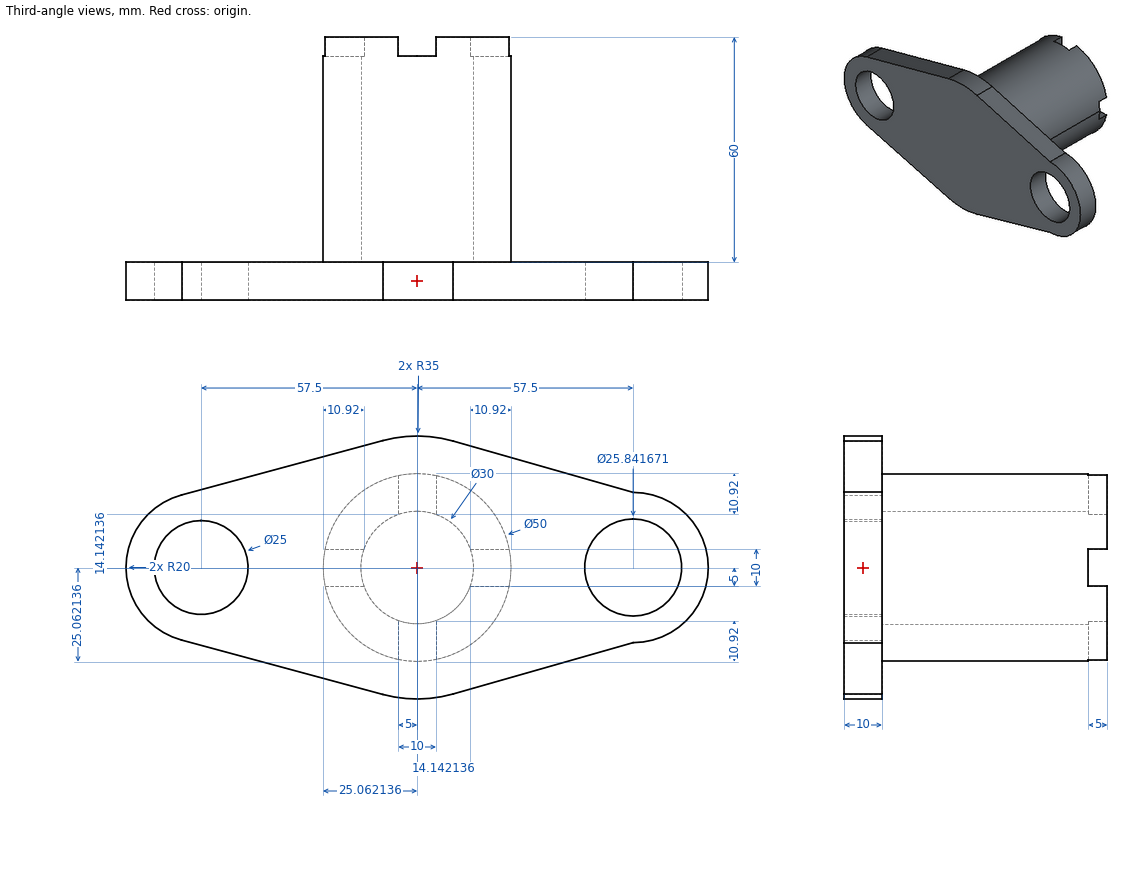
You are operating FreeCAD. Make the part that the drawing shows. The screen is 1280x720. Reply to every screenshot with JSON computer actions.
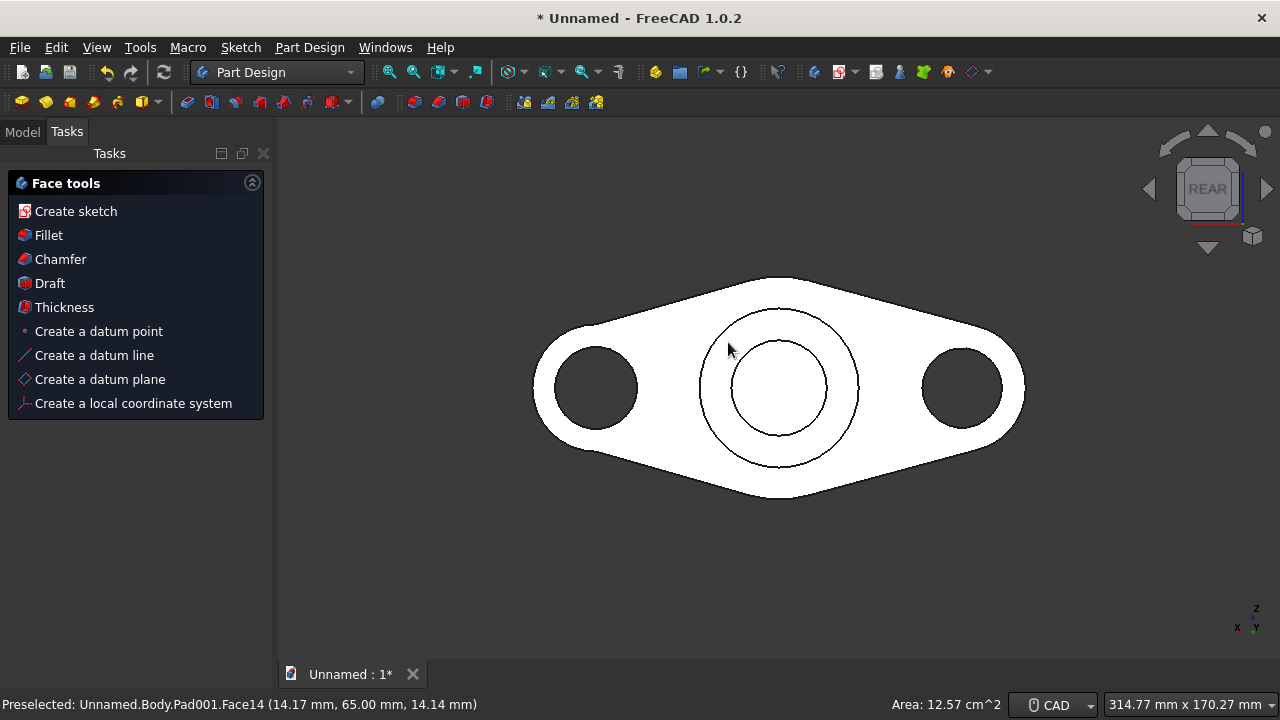
{"action": "left_click", "coordinate": [840, 72]}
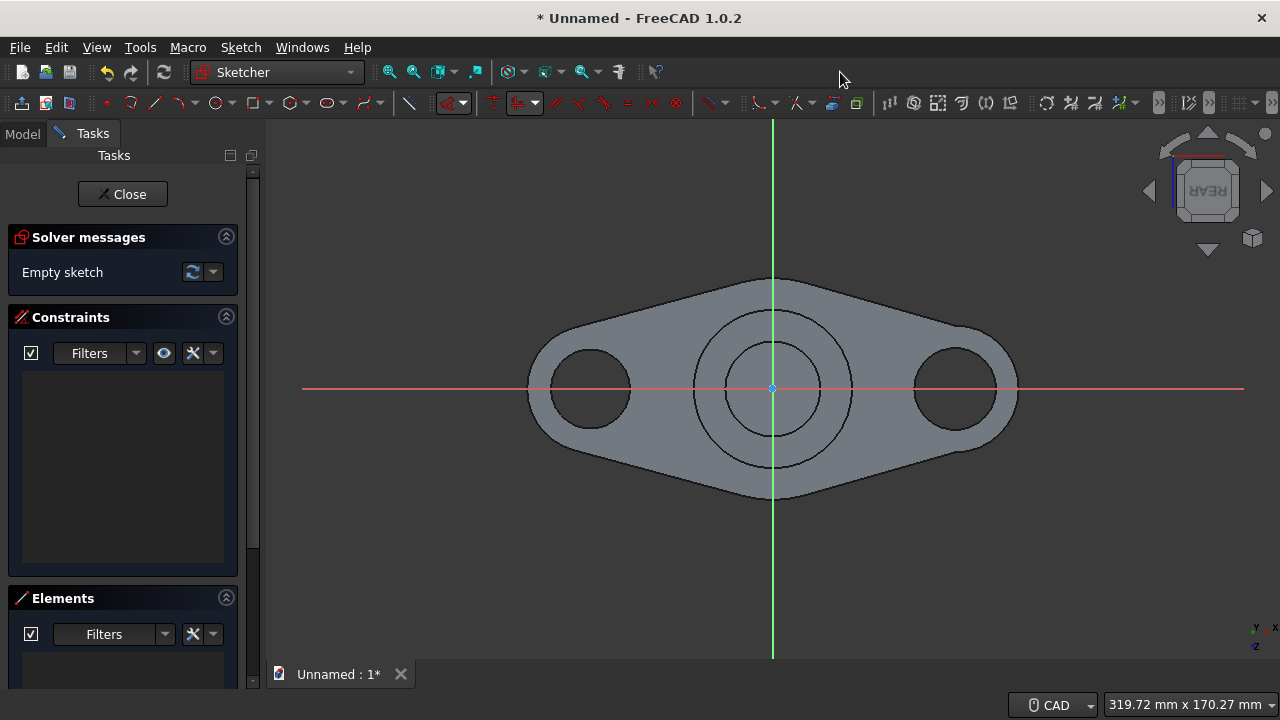
{"action": "scroll", "coordinate": [829, 389], "scroll_direction": "up", "scroll_amount": 4}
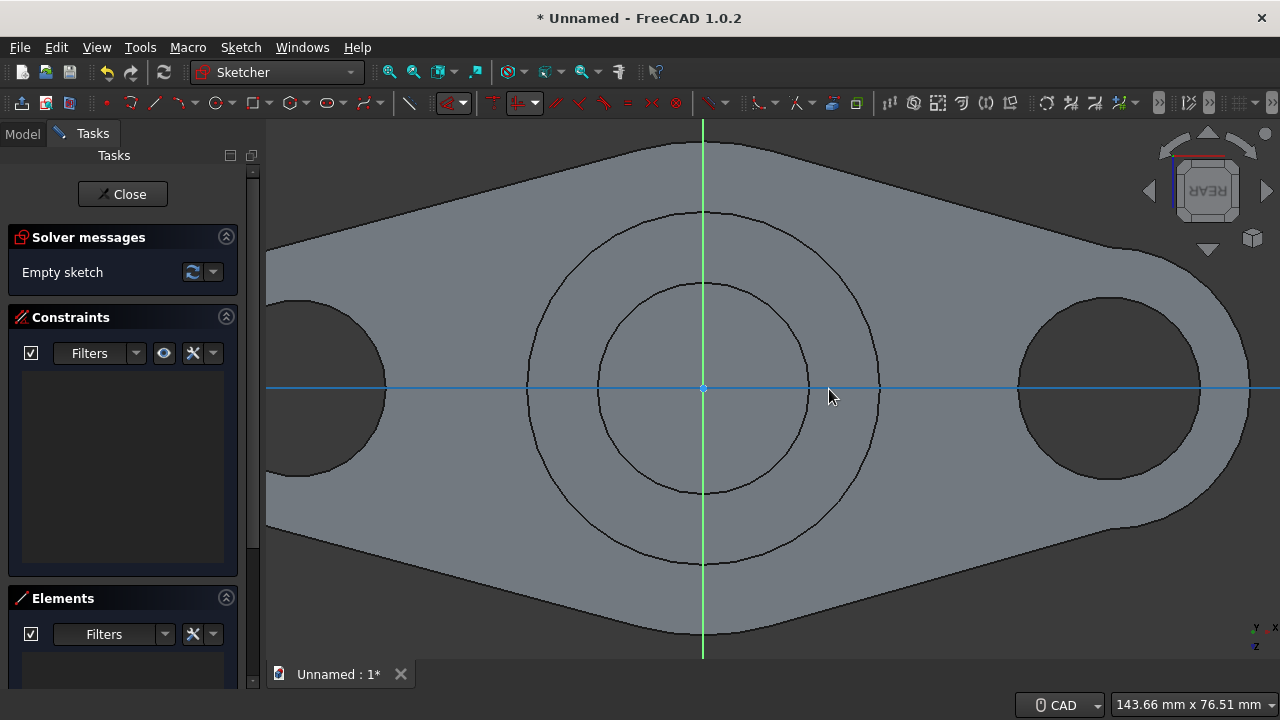
{"action": "left_click", "coordinate": [254, 104]}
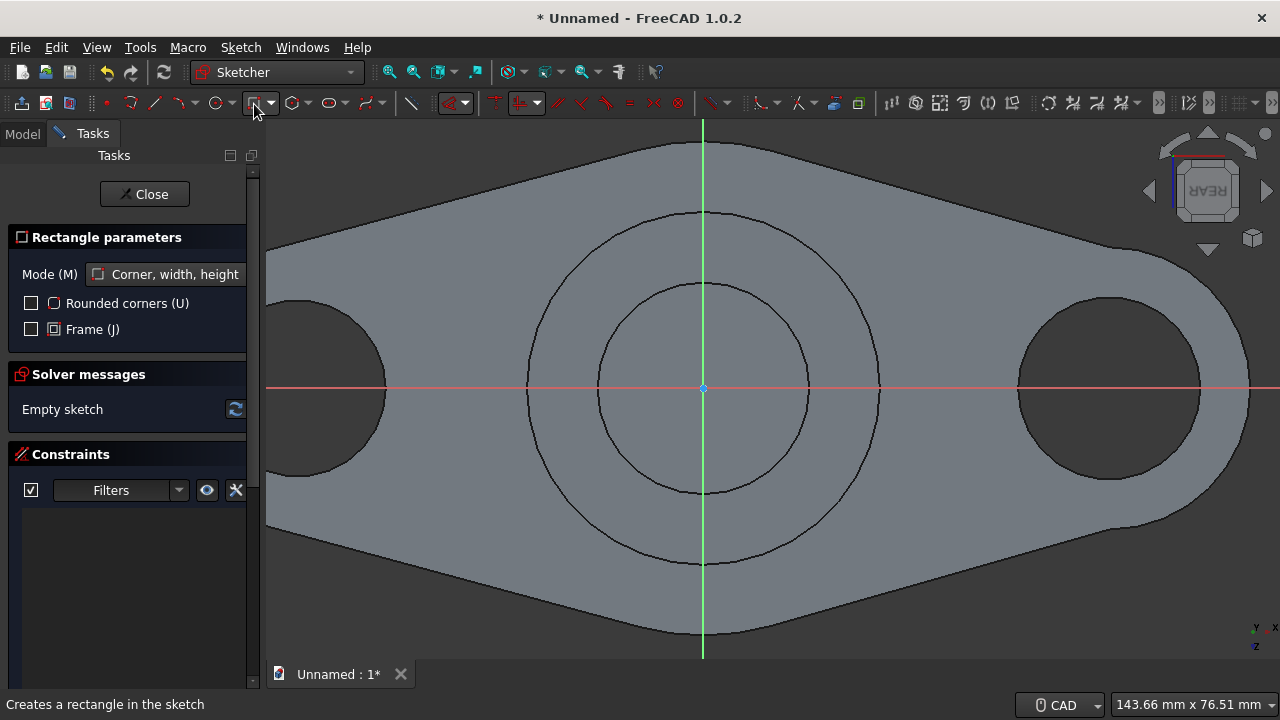
{"action": "left_click", "coordinate": [668, 211]}
{"action": "mouse_move", "coordinate": [739, 289]}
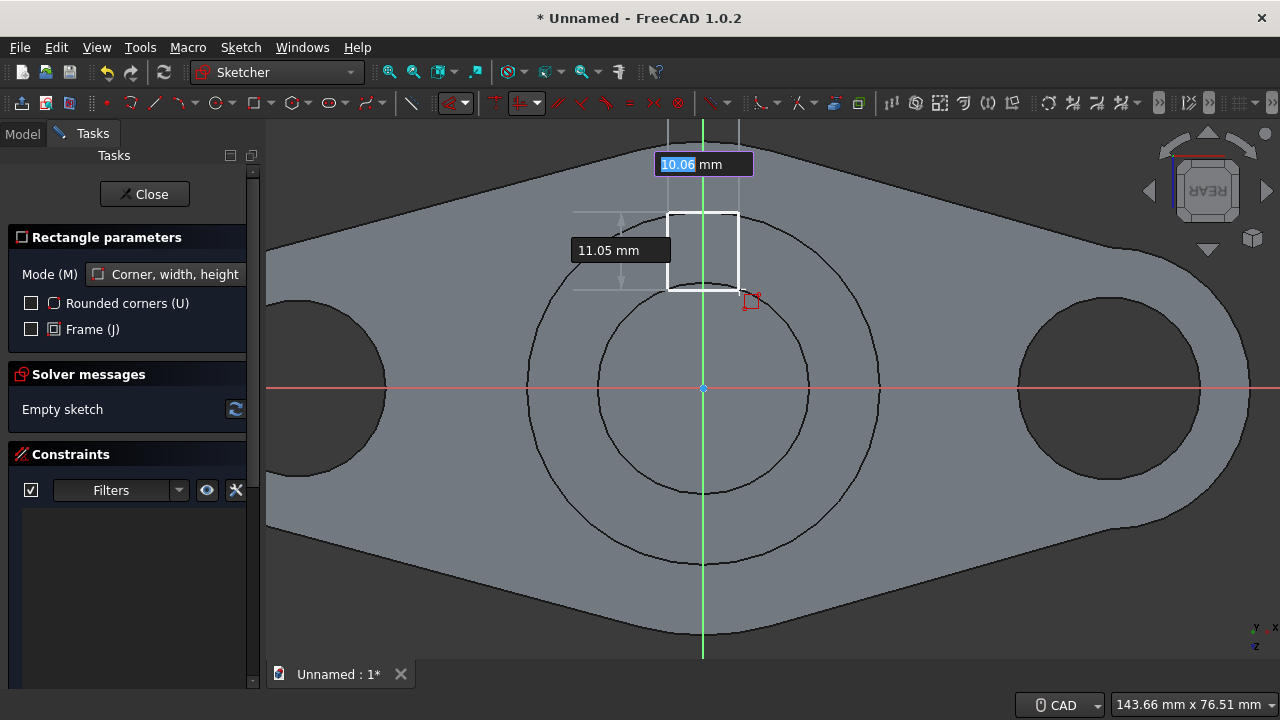
{"action": "type", "text": "10"}
{"action": "key", "text": "Tab"}
{"action": "type", "text": "10.92"}
{"action": "key", "text": "Return"}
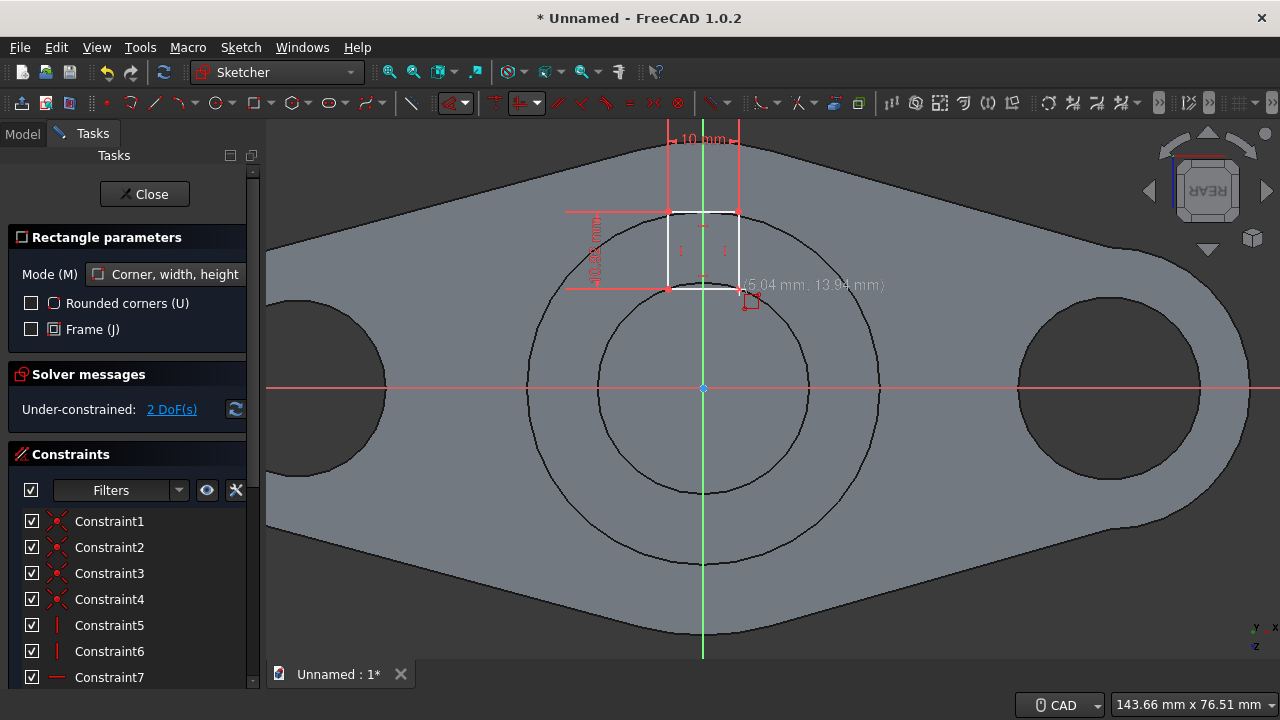
{"action": "left_click", "coordinate": [803, 353]}
{"action": "mouse_move", "coordinate": [880, 424]}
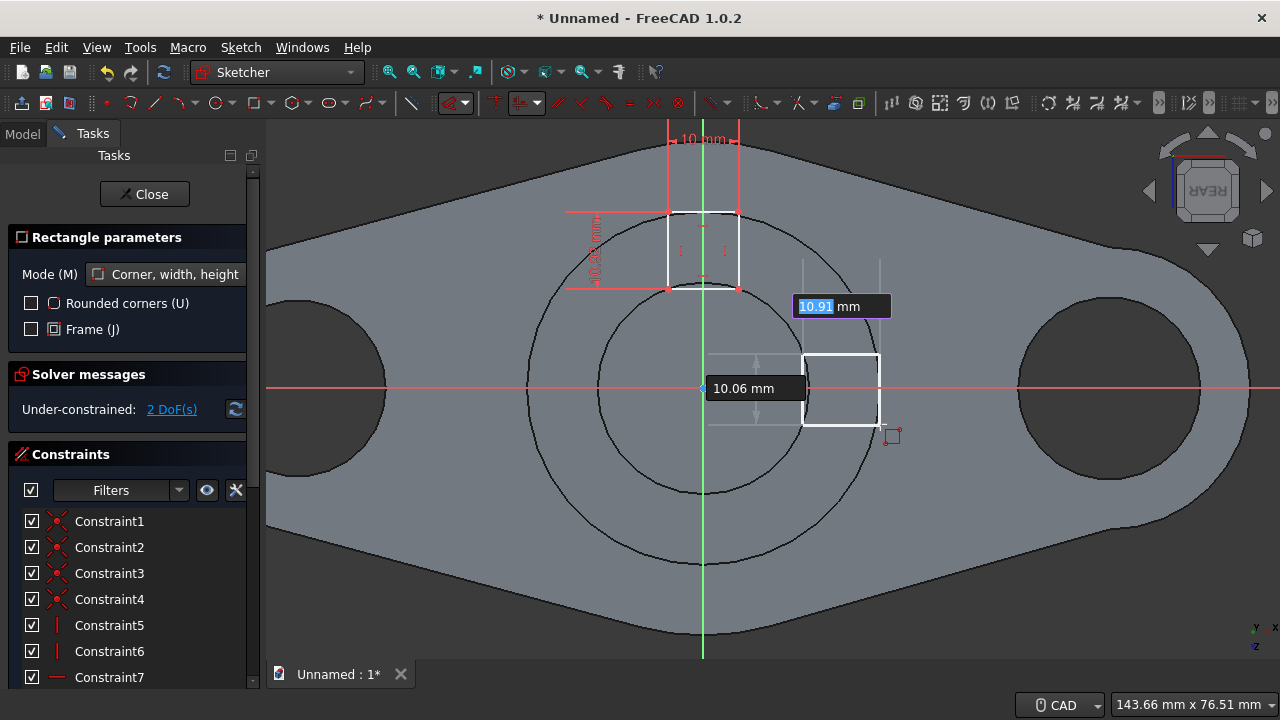
{"action": "type", "text": "10.92"}
{"action": "key", "text": "Tab"}
{"action": "type", "text": "10"}
{"action": "key", "text": "Return"}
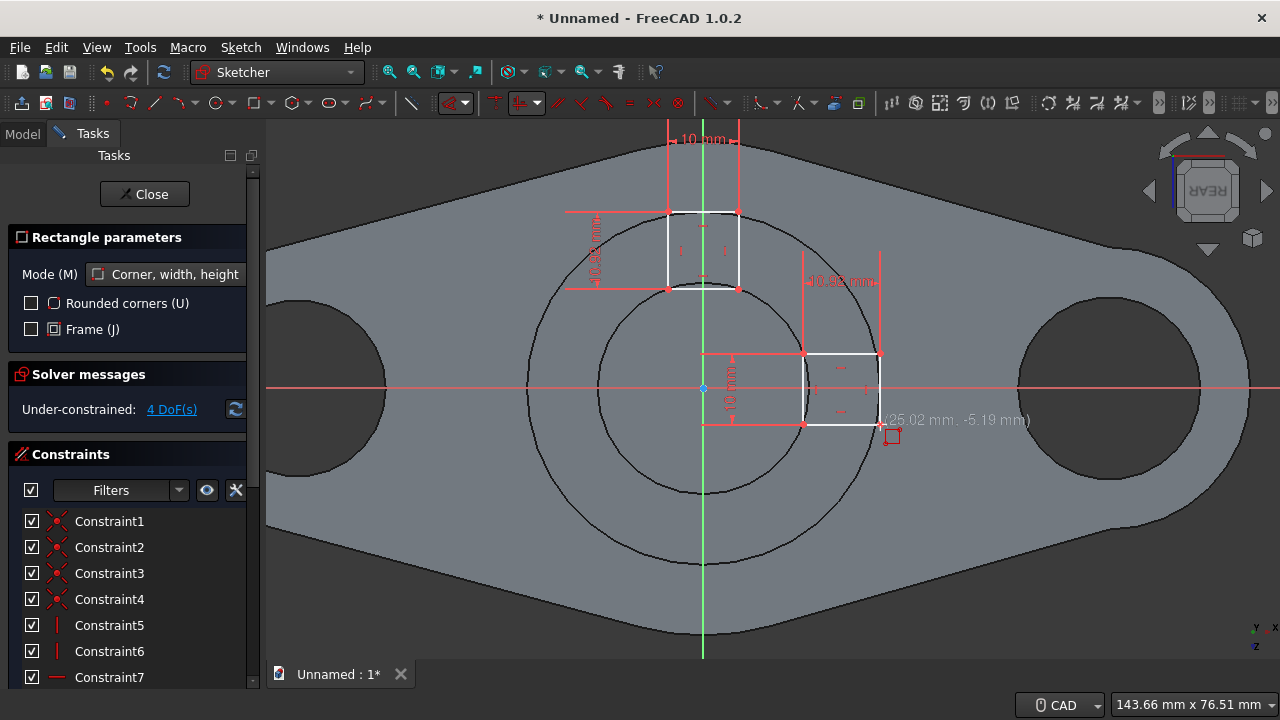
{"action": "left_click", "coordinate": [668, 488]}
{"action": "mouse_move", "coordinate": [739, 565]}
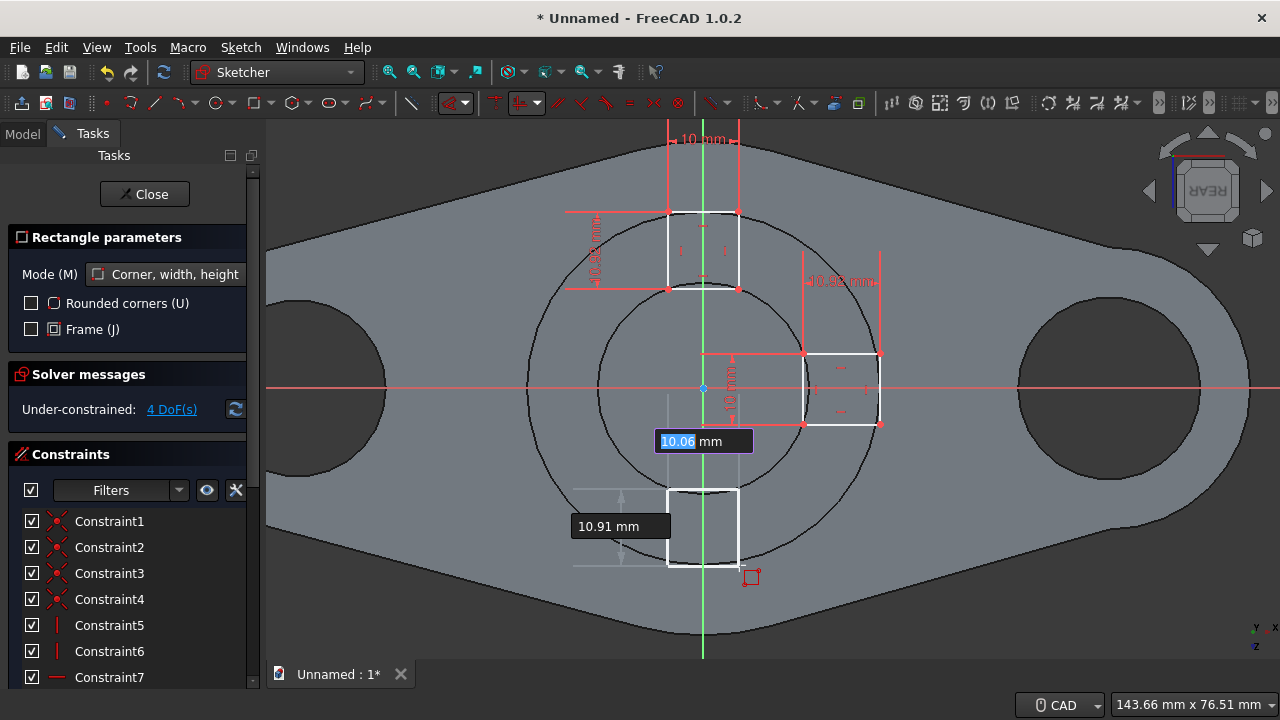
{"action": "type", "text": "10"}
{"action": "key", "text": "Tab"}
{"action": "type", "text": "10.92"}
{"action": "key", "text": "Return"}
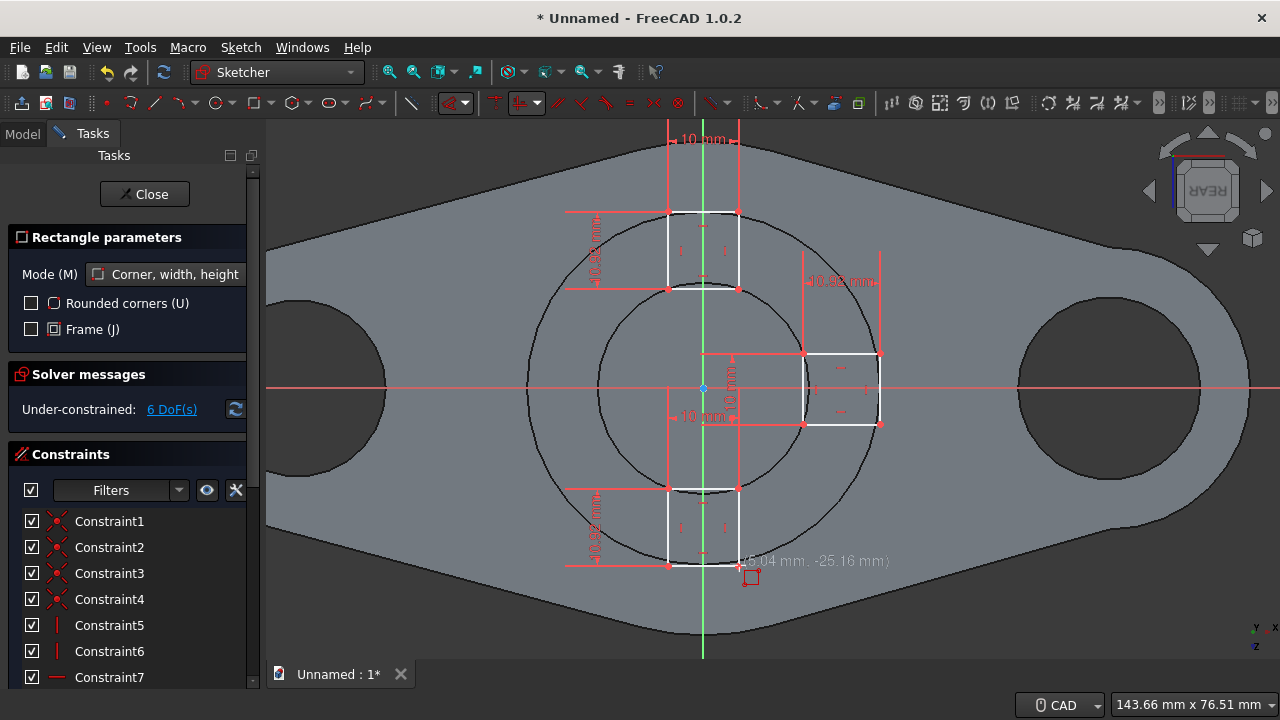
{"action": "left_click", "coordinate": [527, 353]}
{"action": "mouse_move", "coordinate": [604, 424]}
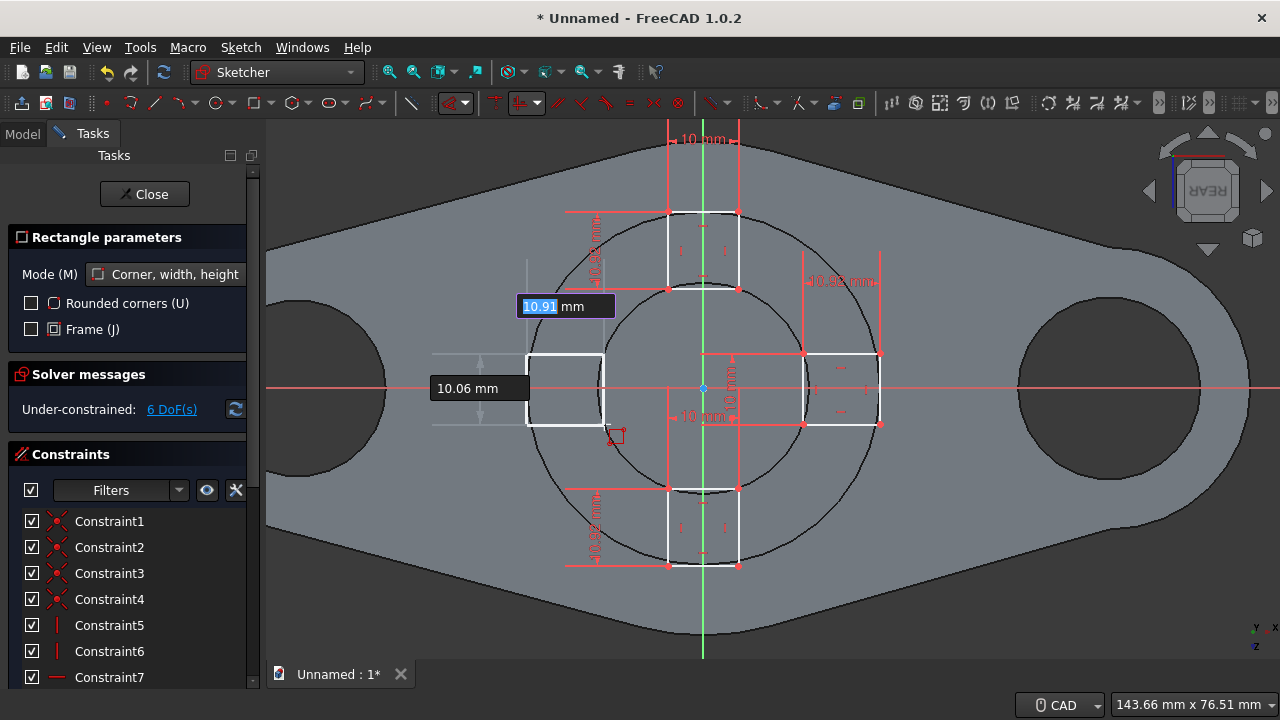
{"action": "type", "text": "10.92"}
{"action": "key", "text": "Tab"}
{"action": "type", "text": "10"}
{"action": "key", "text": "Return"}
{"action": "key", "text": "Escape"}